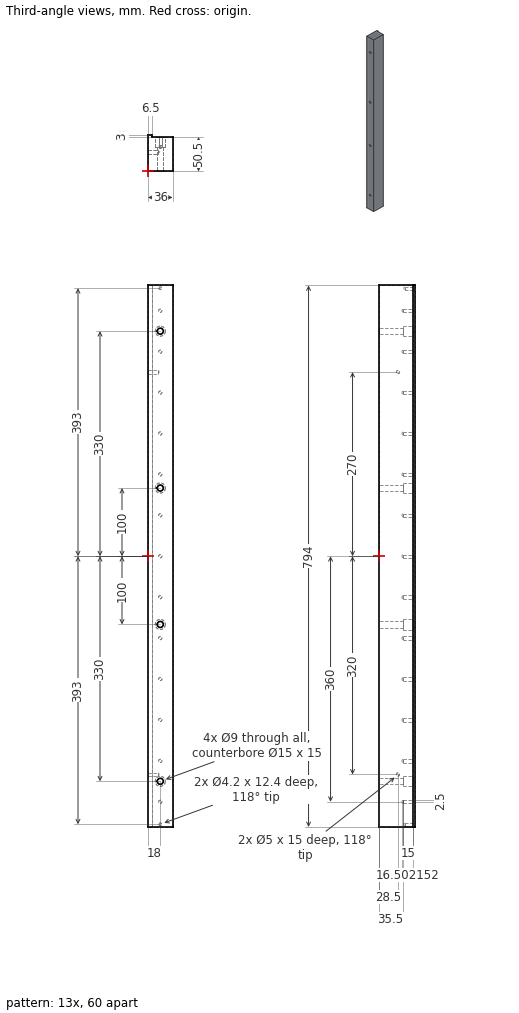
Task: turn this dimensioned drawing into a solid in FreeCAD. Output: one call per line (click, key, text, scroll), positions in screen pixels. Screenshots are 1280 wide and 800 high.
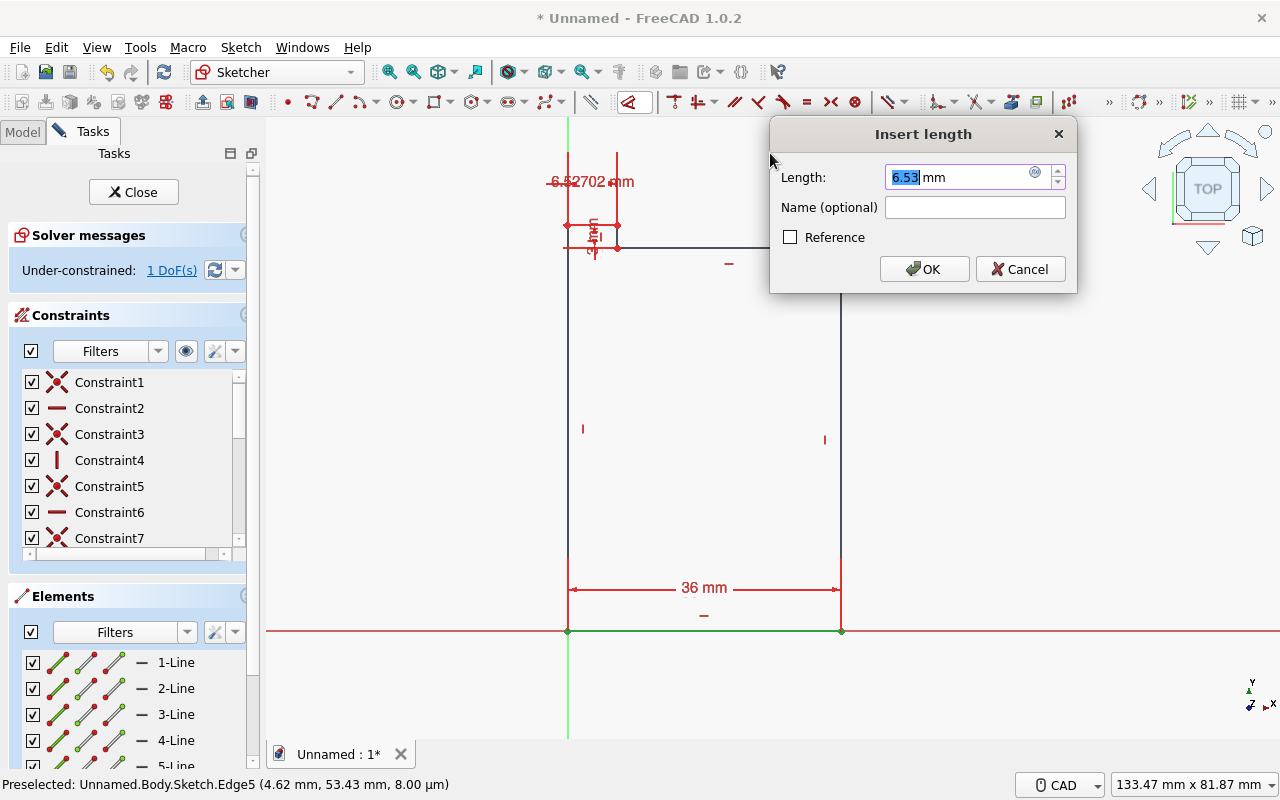
text(6.5)
key(Return)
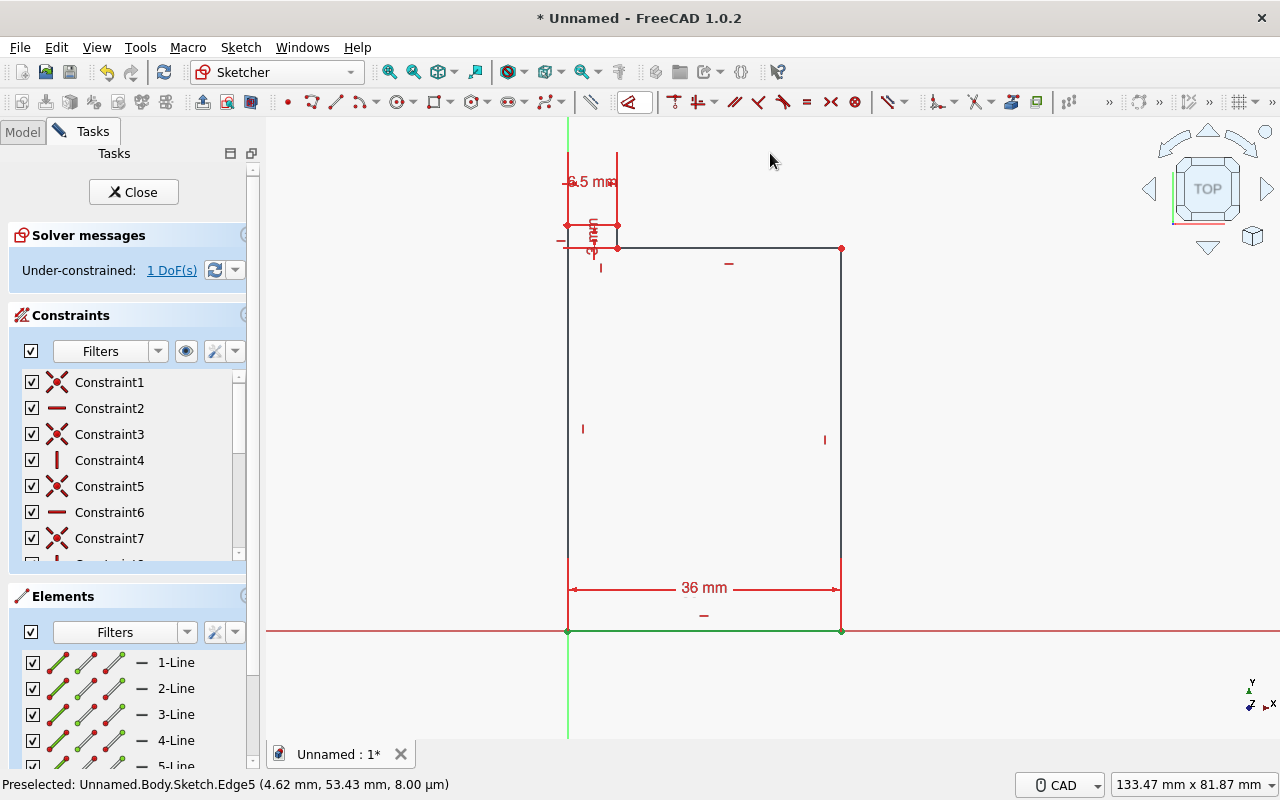
click(841, 516)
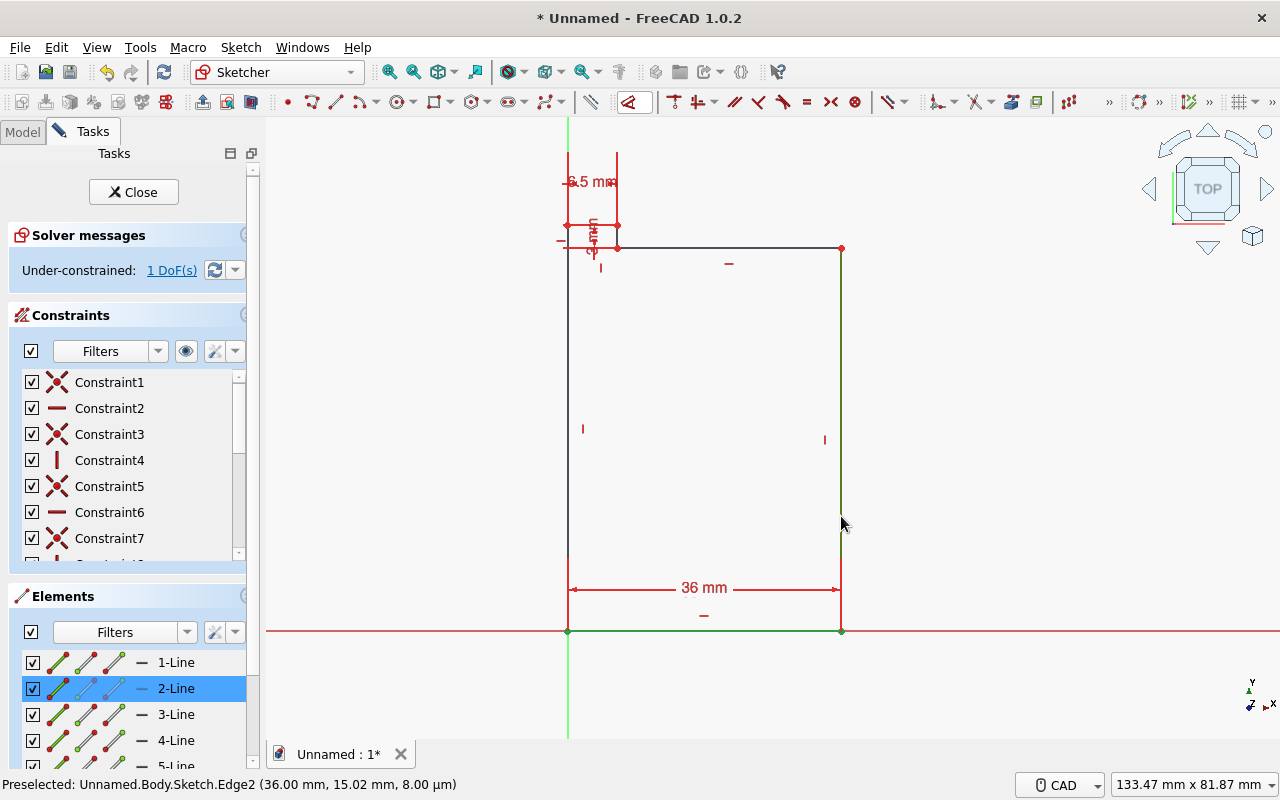
click(646, 102)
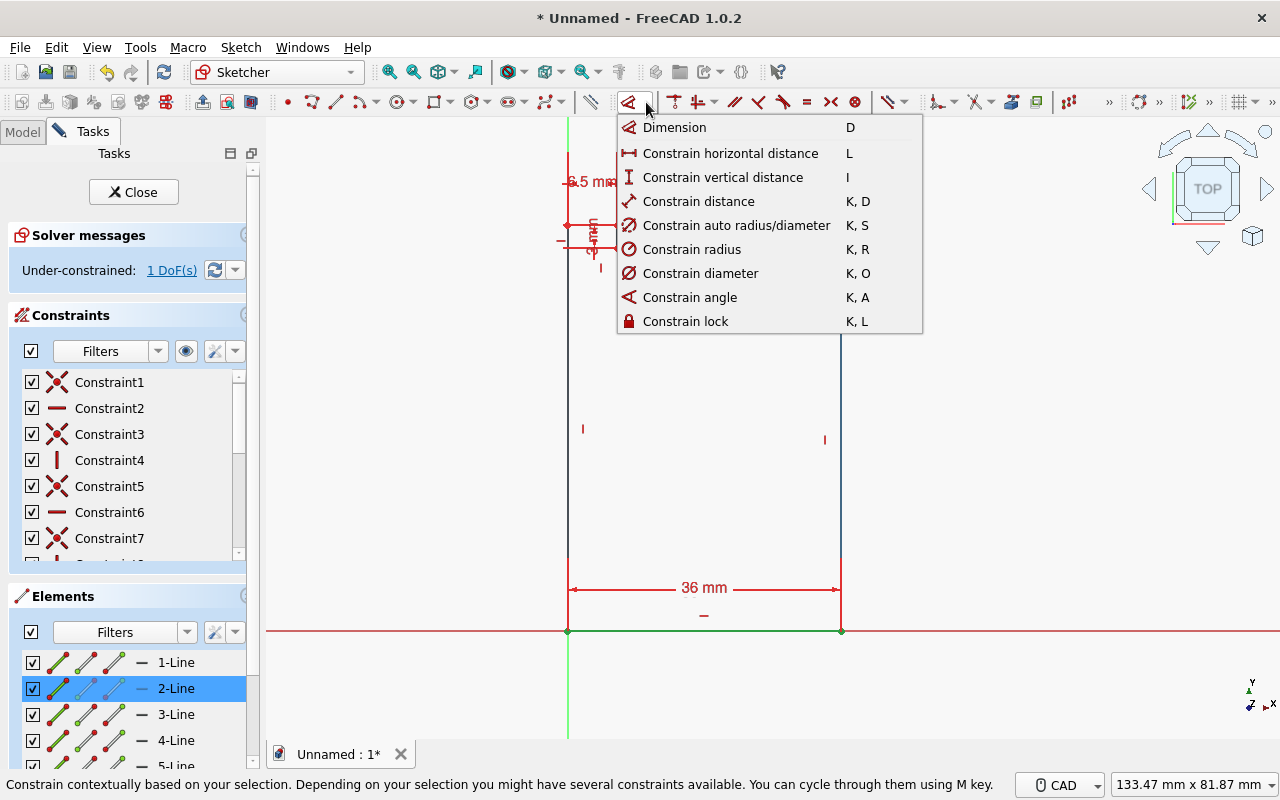
click(770, 177)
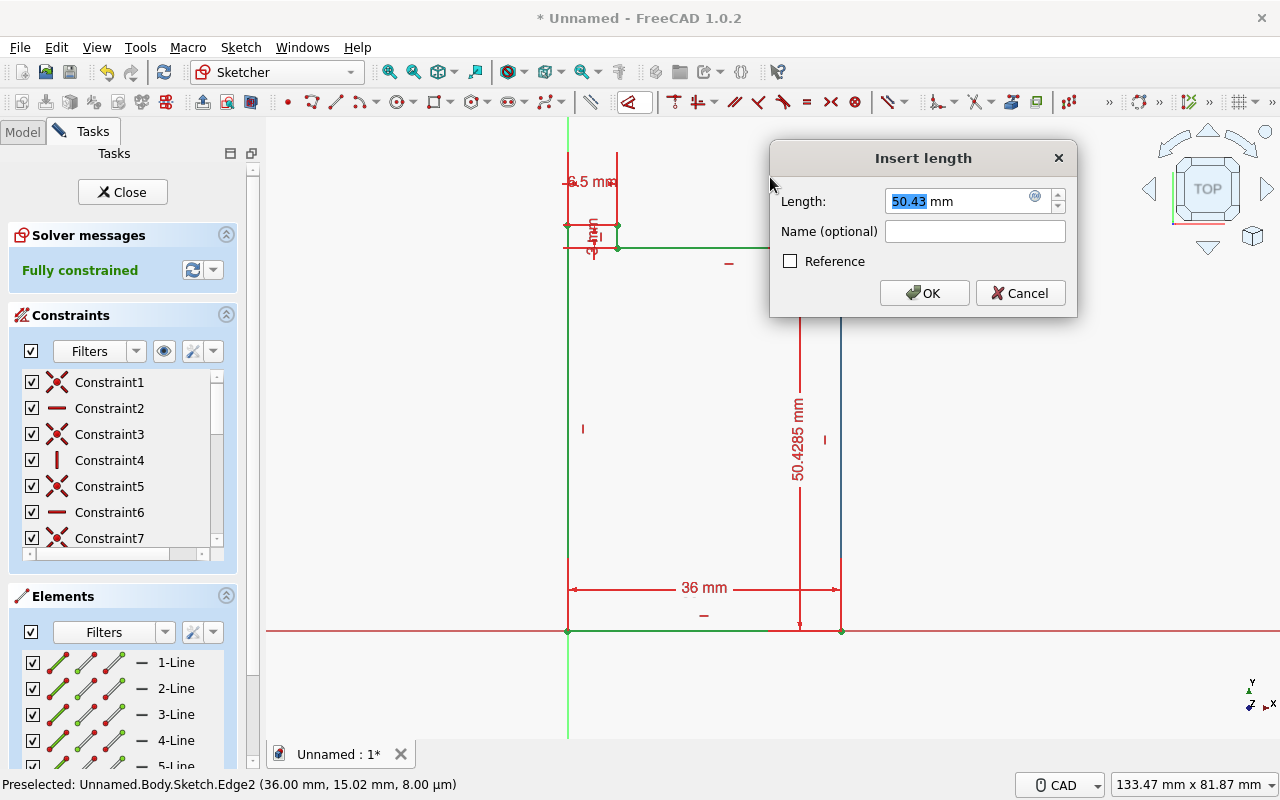
text(50.5)
key(Return)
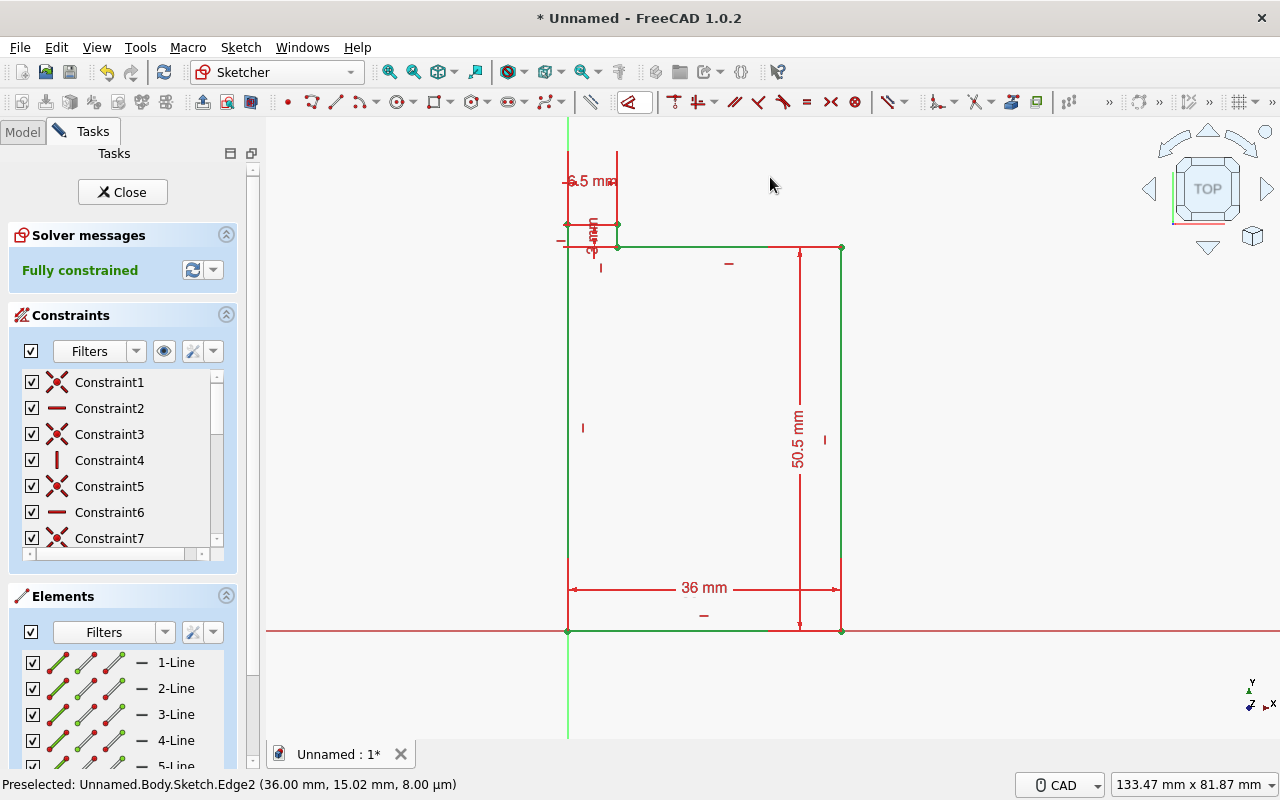
click(123, 192)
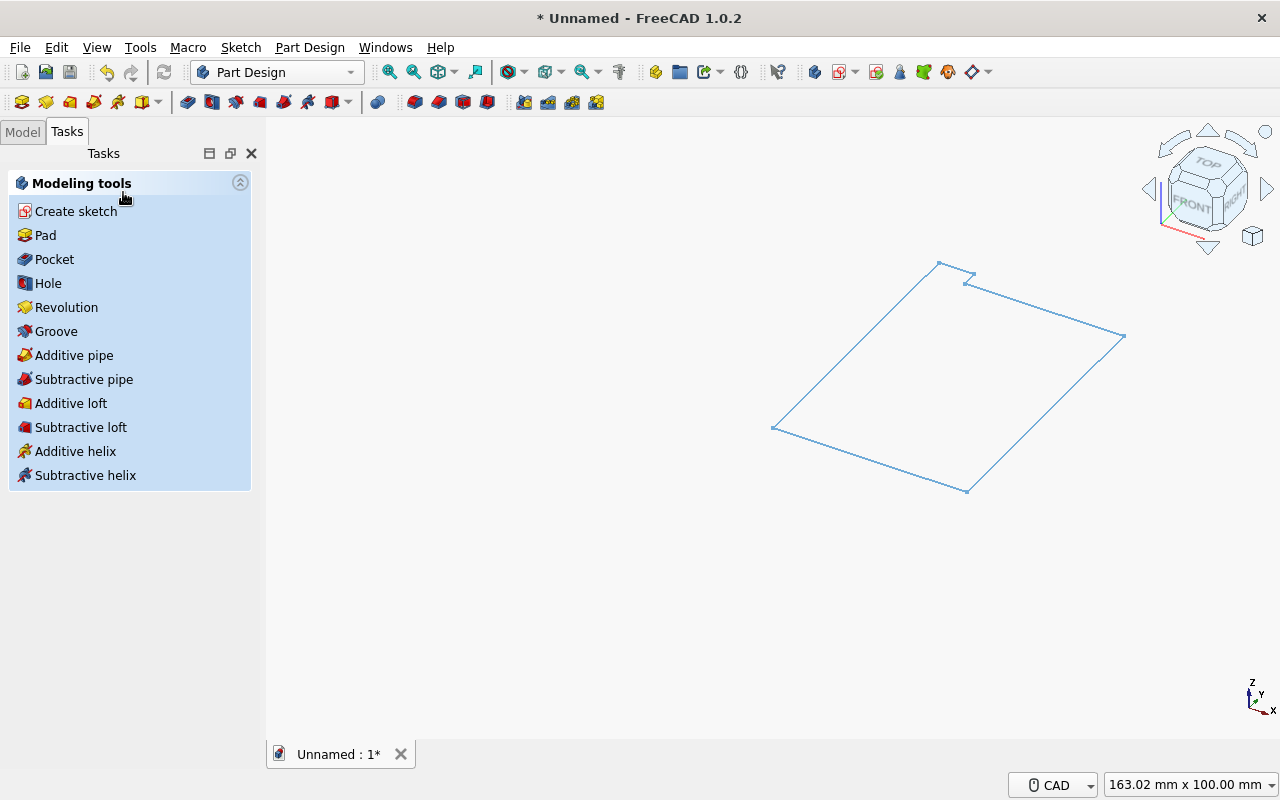
click(22, 102)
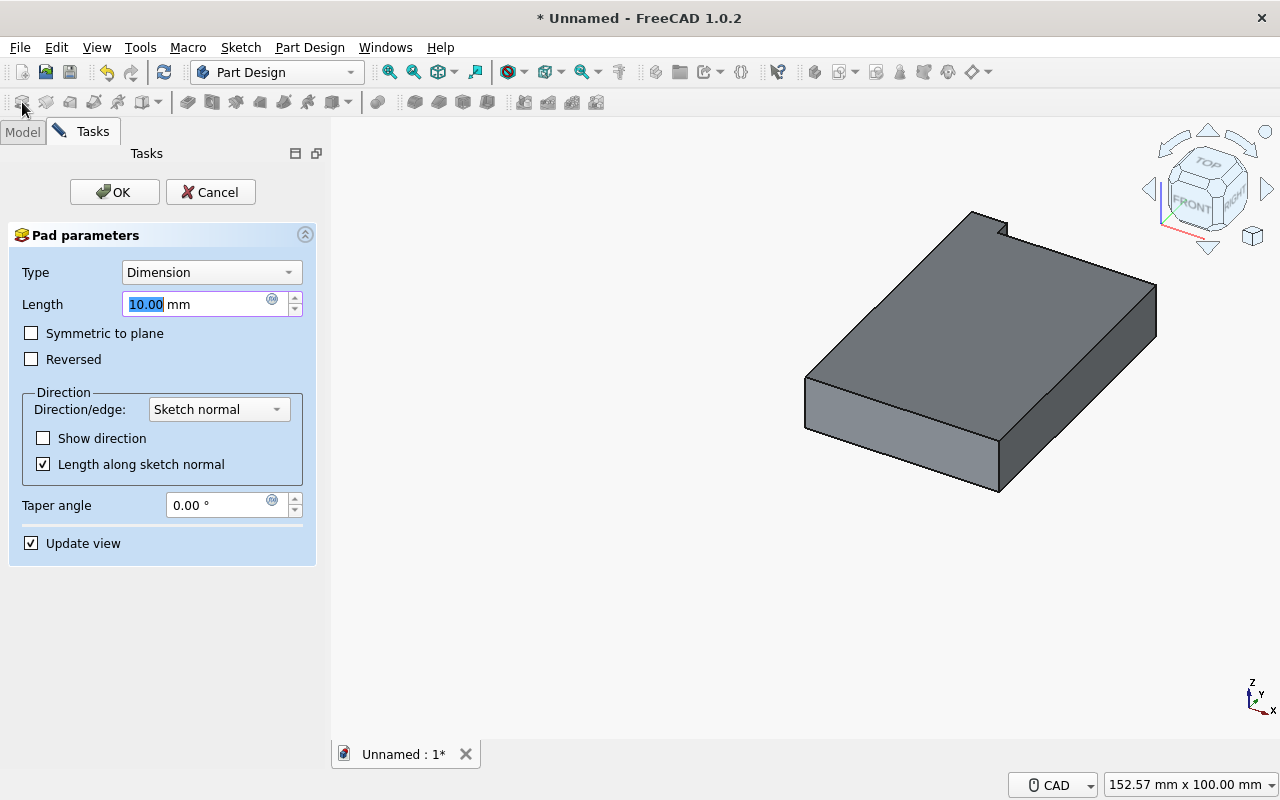
text(794)
key(Tab)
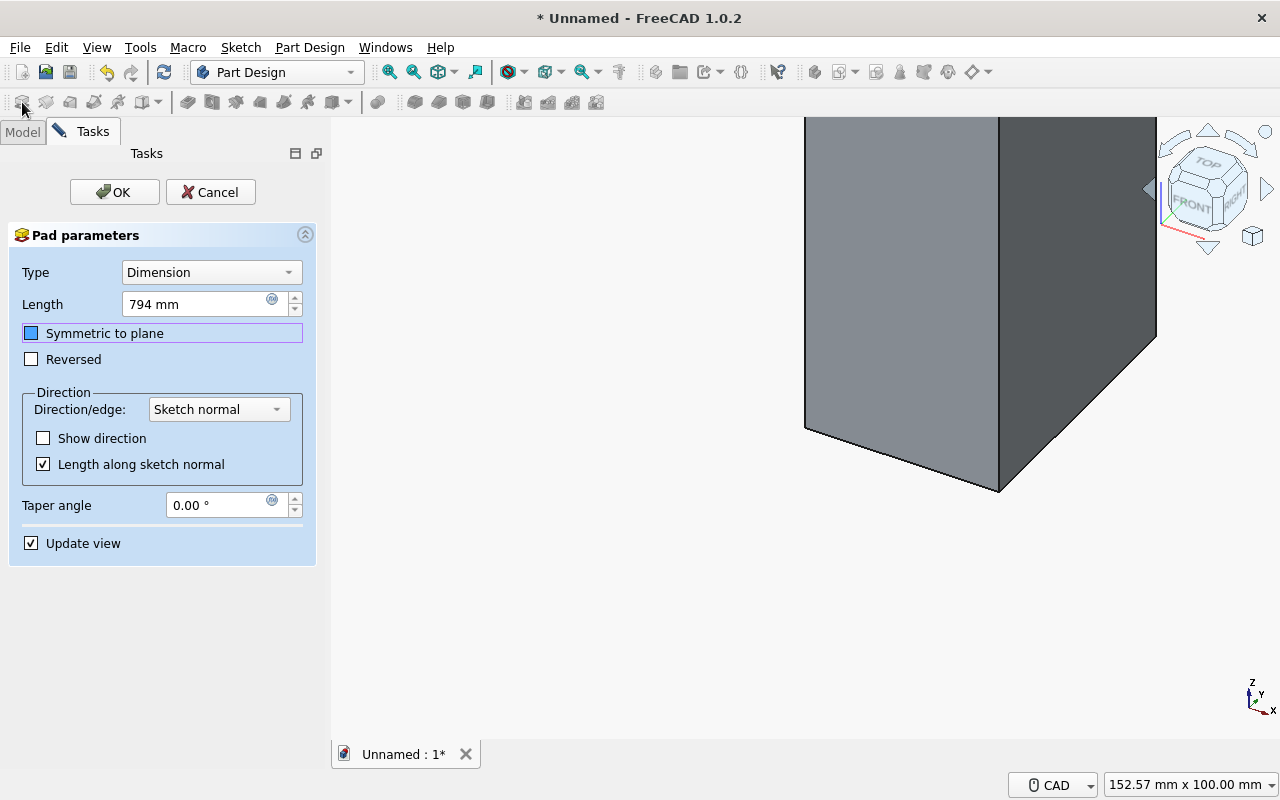
click(30, 333)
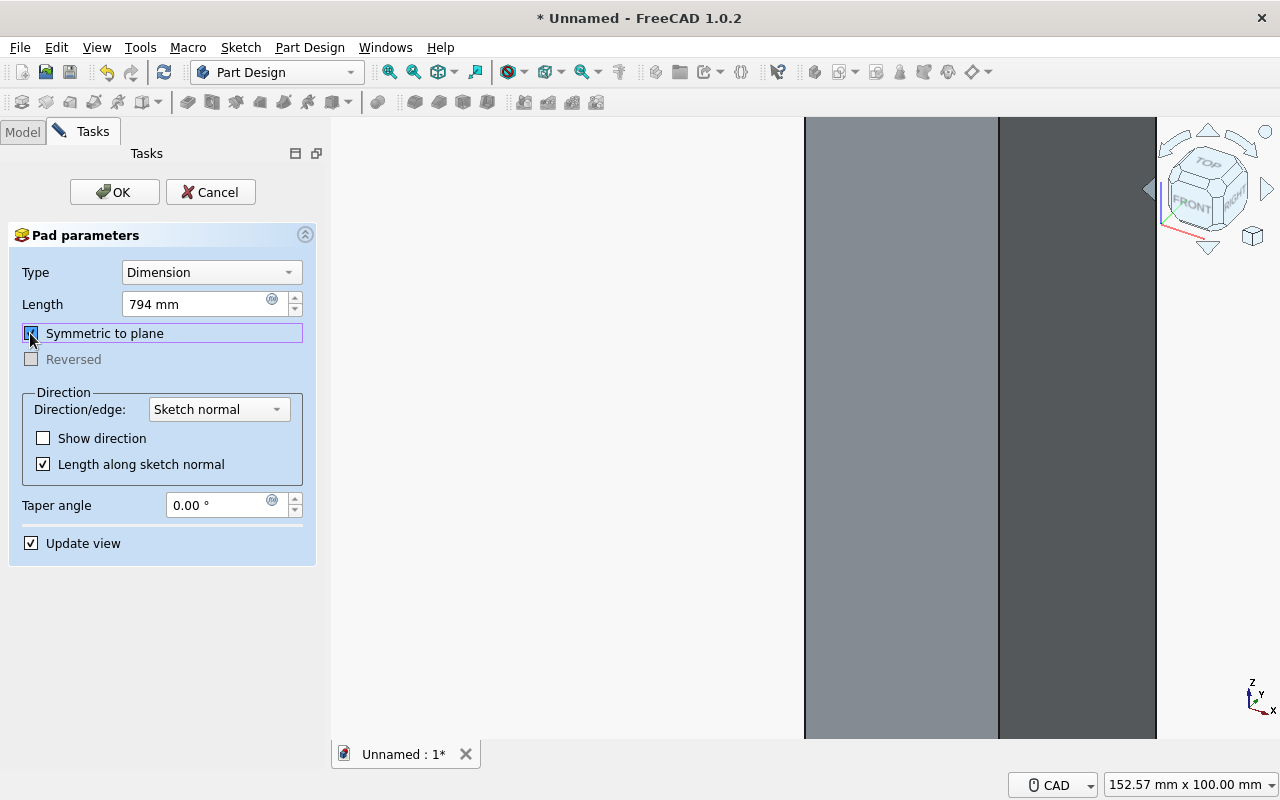
click(115, 192)